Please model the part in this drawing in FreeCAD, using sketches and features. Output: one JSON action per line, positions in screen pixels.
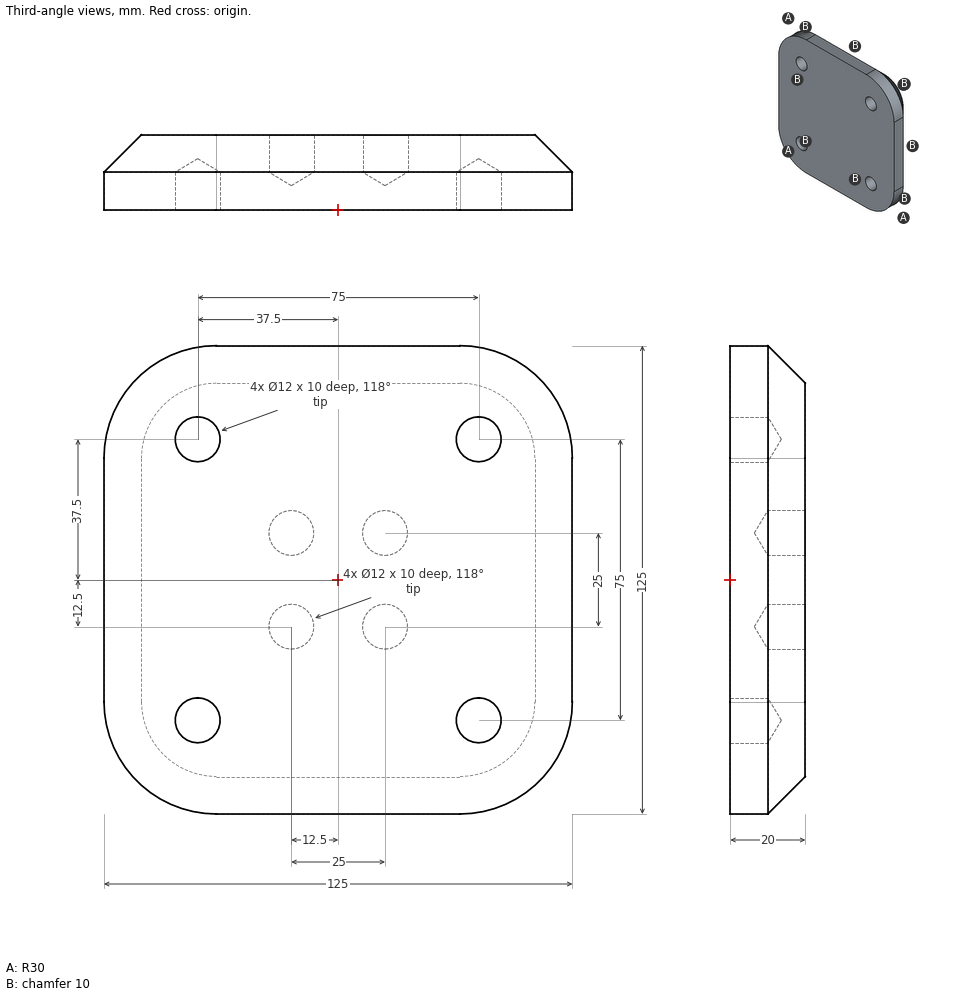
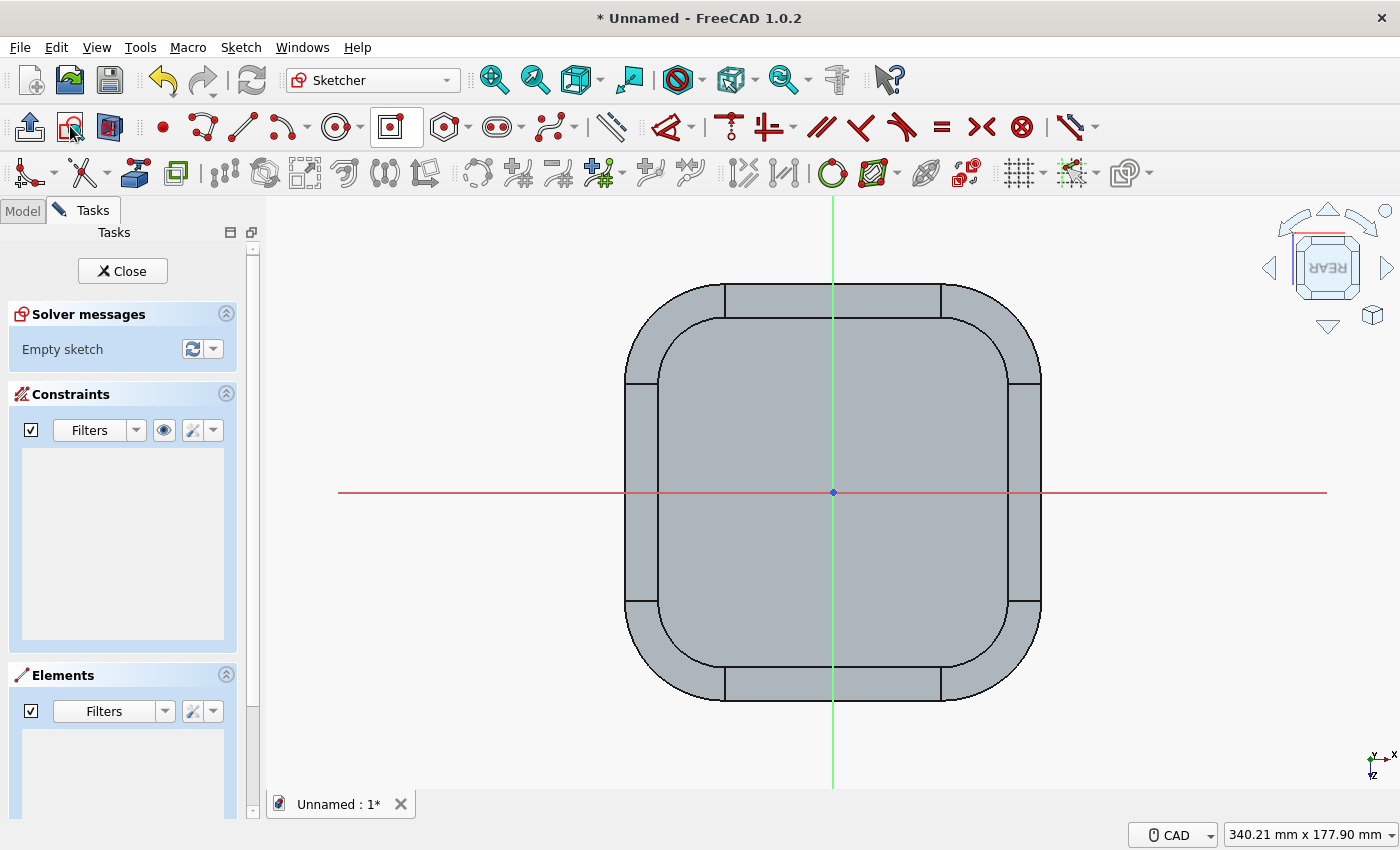
{"action": "scroll", "coordinate": [863, 493], "scroll_direction": "up", "scroll_amount": 6}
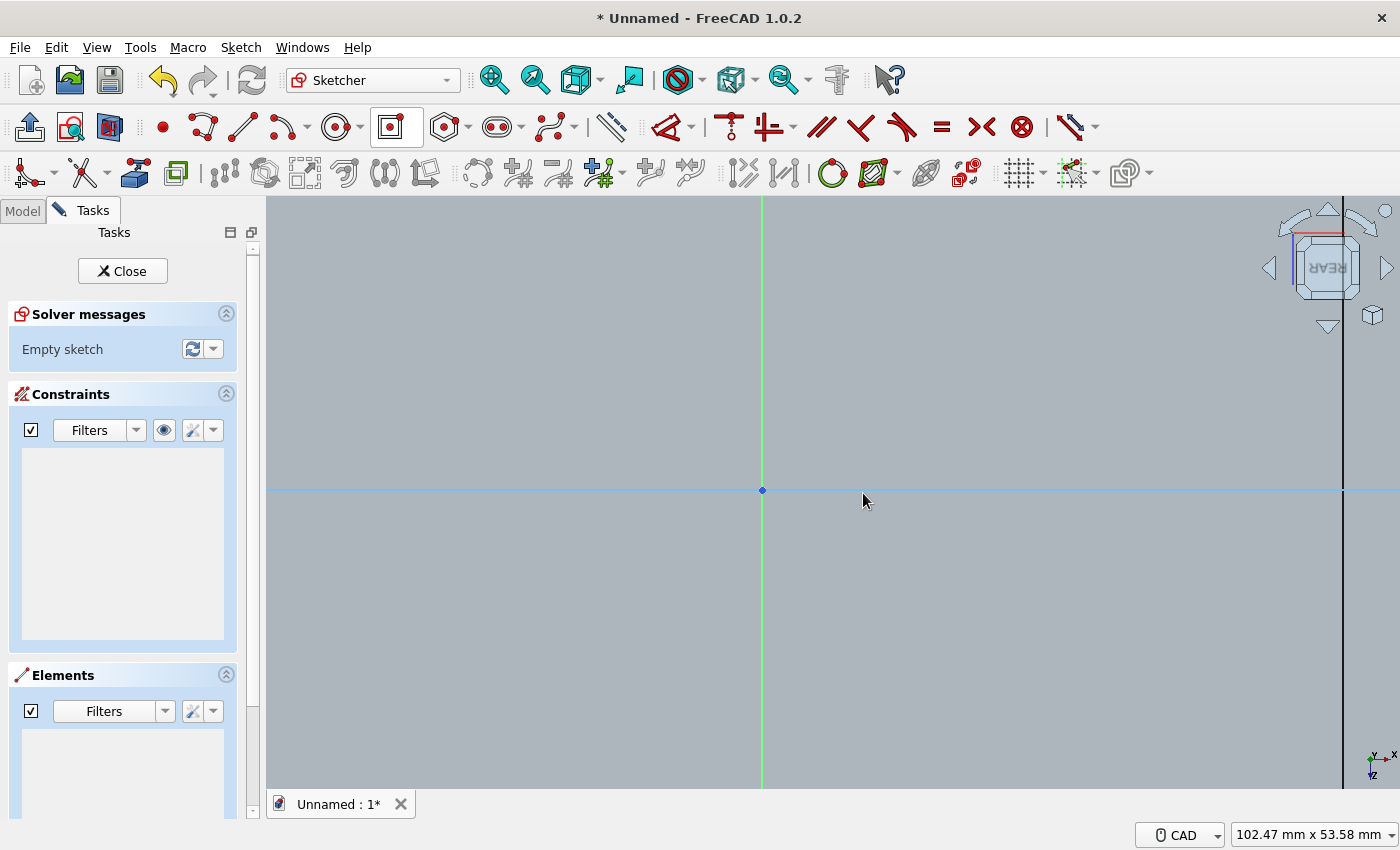
{"action": "key", "text": "g c"}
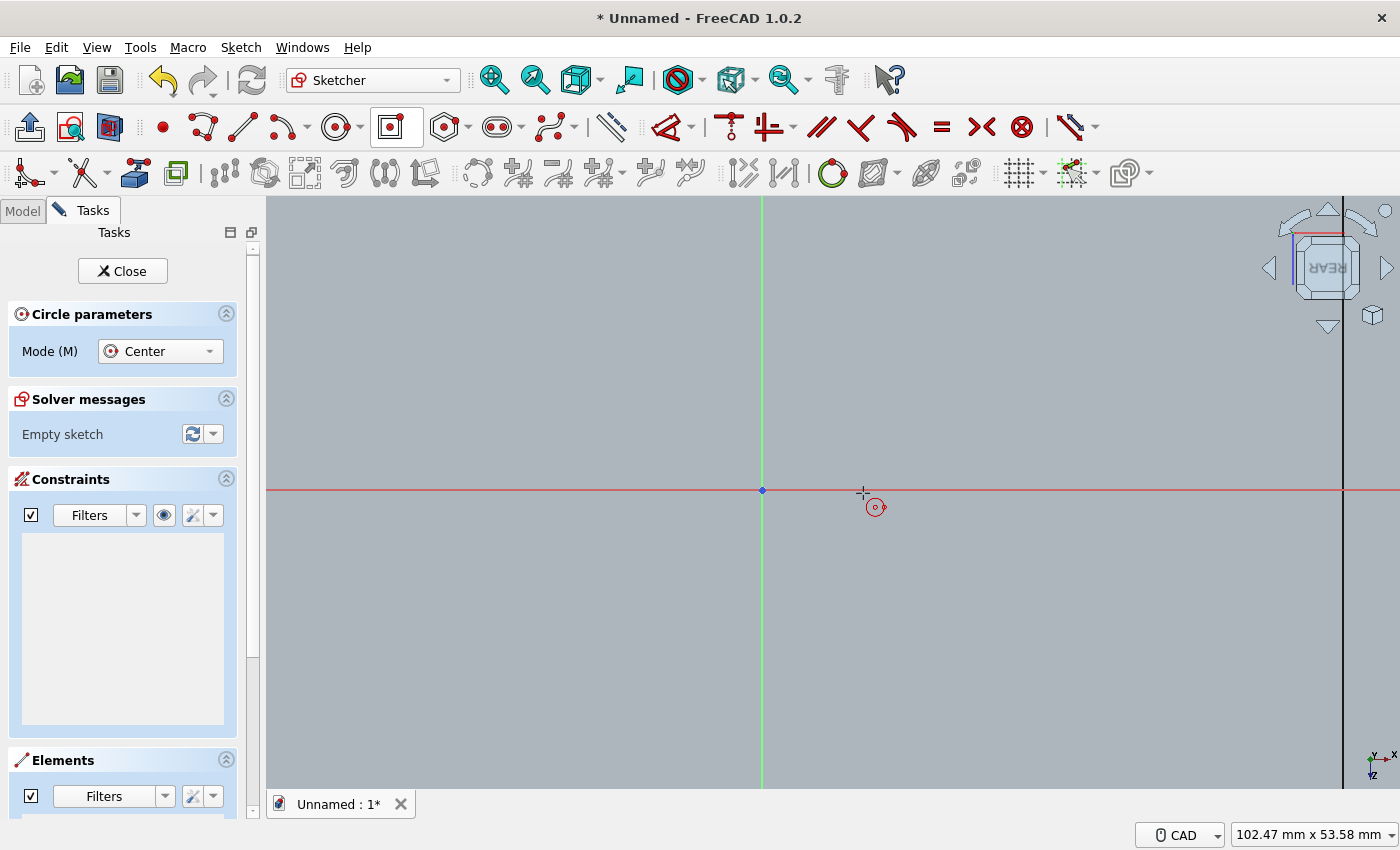
{"action": "left_click", "coordinate": [624, 352]}
{"action": "left_click", "coordinate": [671, 305]}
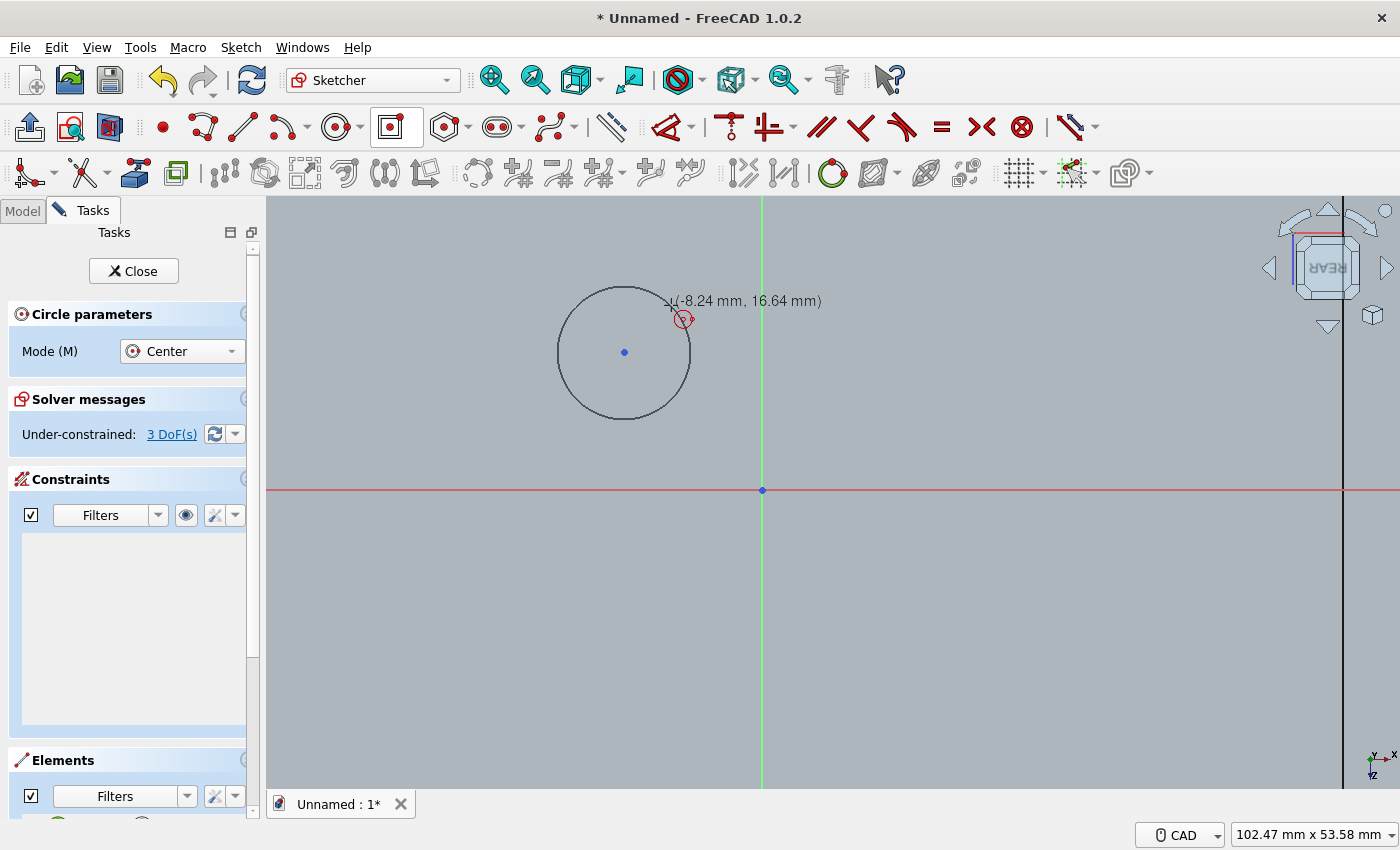
{"action": "left_click", "coordinate": [901, 352]}
{"action": "left_click", "coordinate": [947, 305]}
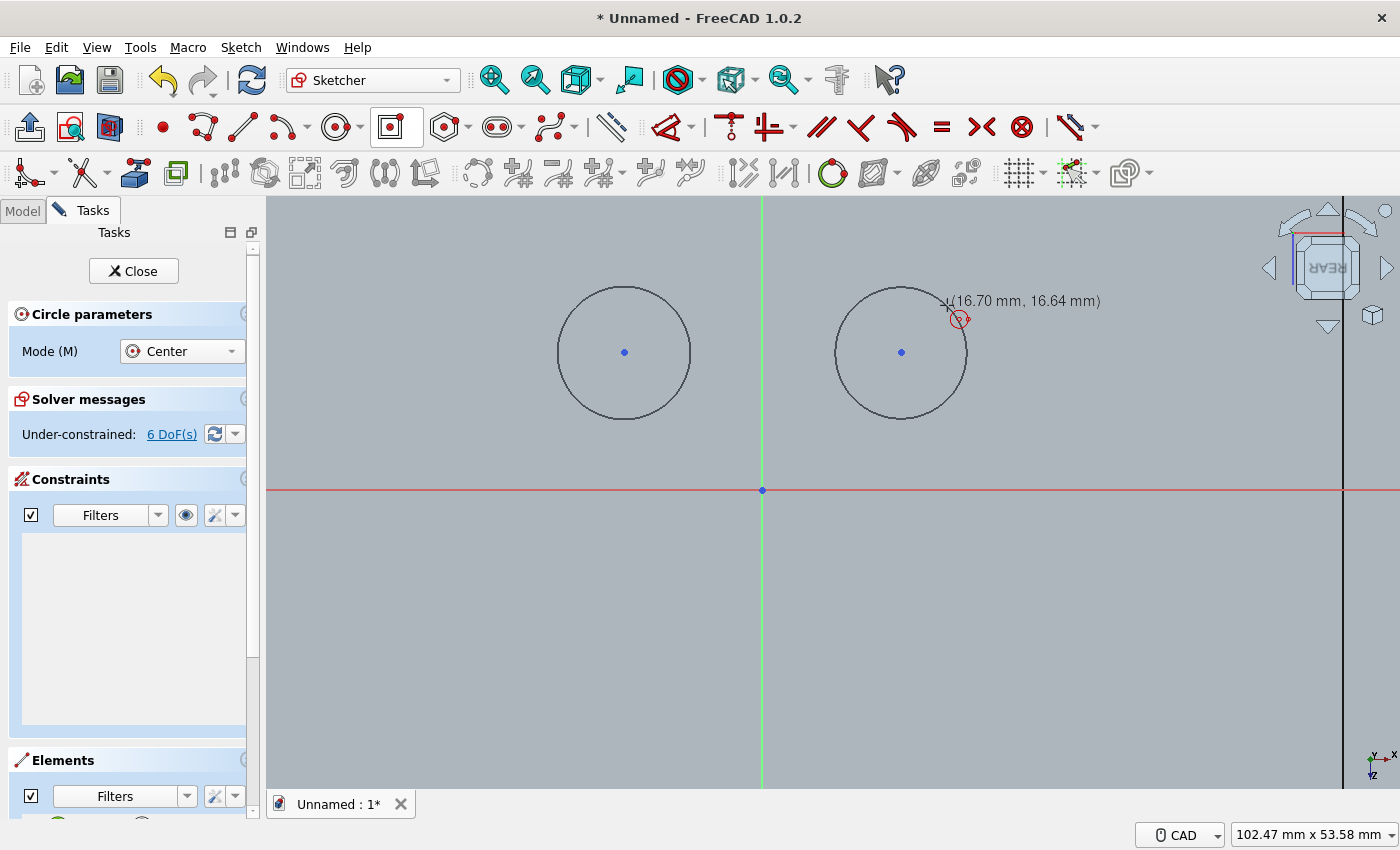
{"action": "left_click", "coordinate": [901, 629]}
{"action": "left_click", "coordinate": [947, 582]}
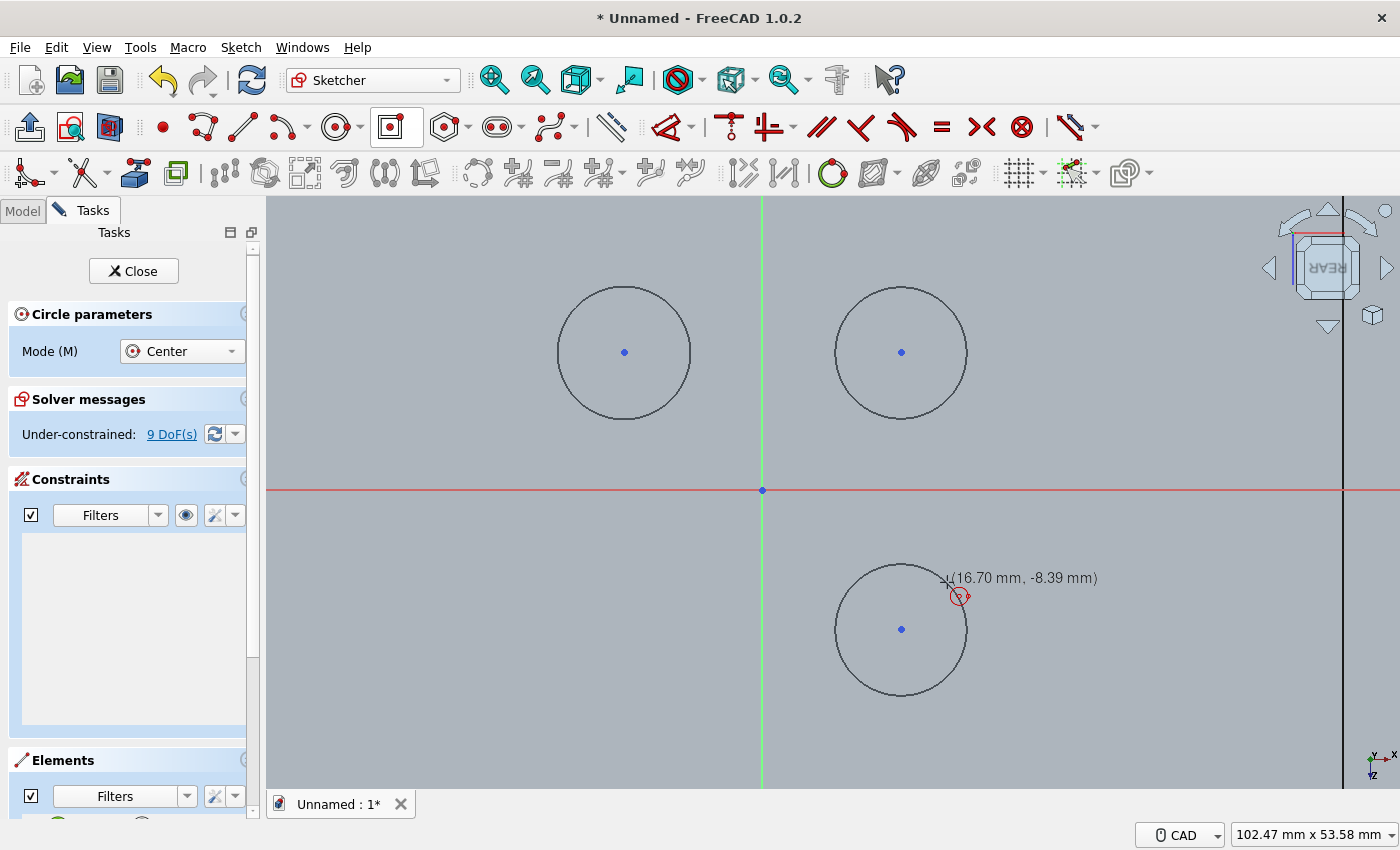
{"action": "left_click", "coordinate": [624, 629]}
{"action": "left_click", "coordinate": [671, 582]}
{"action": "key", "text": "Escape"}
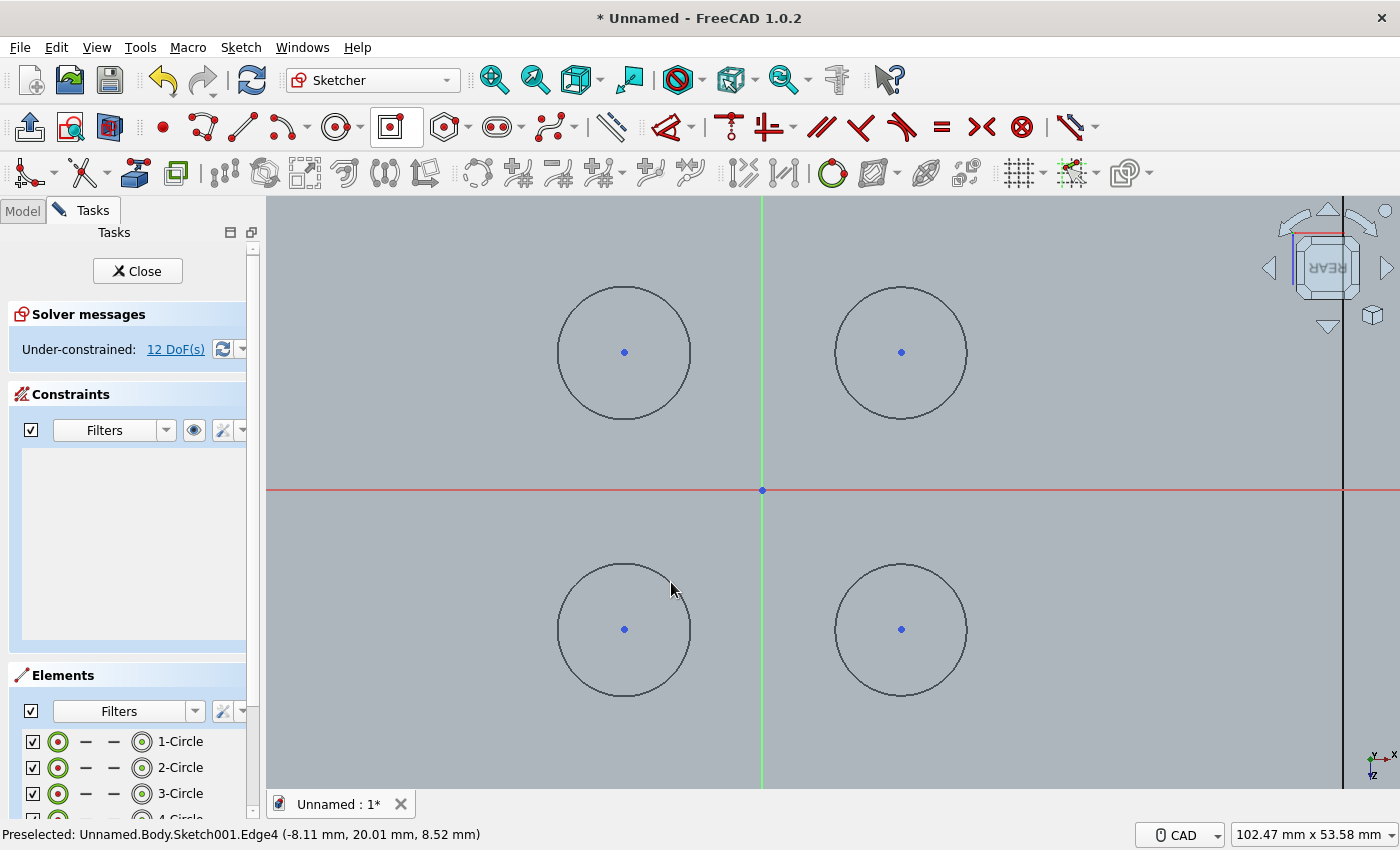
{"action": "left_click", "coordinate": [671, 306]}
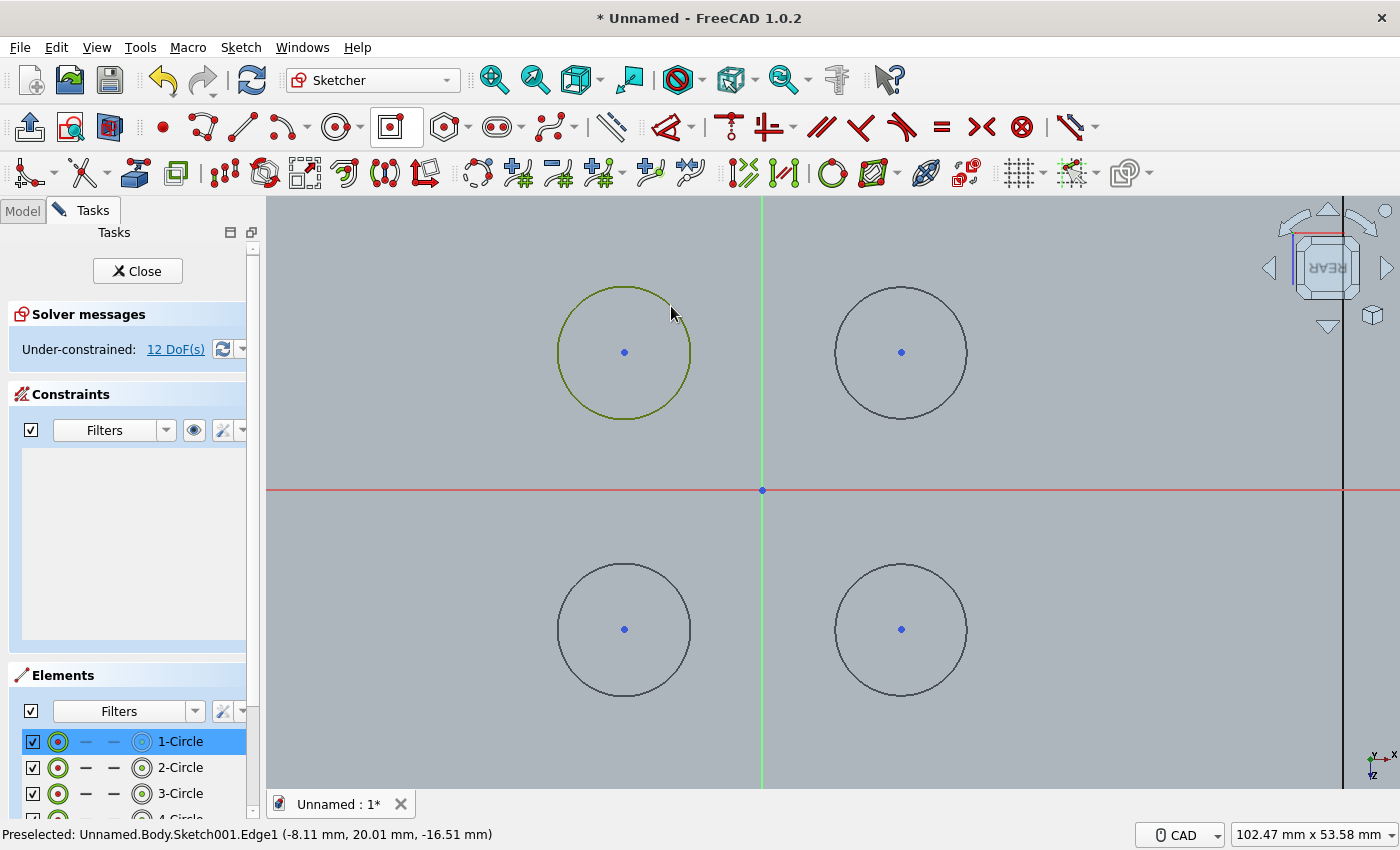
{"action": "left_click", "coordinate": [947, 306]}